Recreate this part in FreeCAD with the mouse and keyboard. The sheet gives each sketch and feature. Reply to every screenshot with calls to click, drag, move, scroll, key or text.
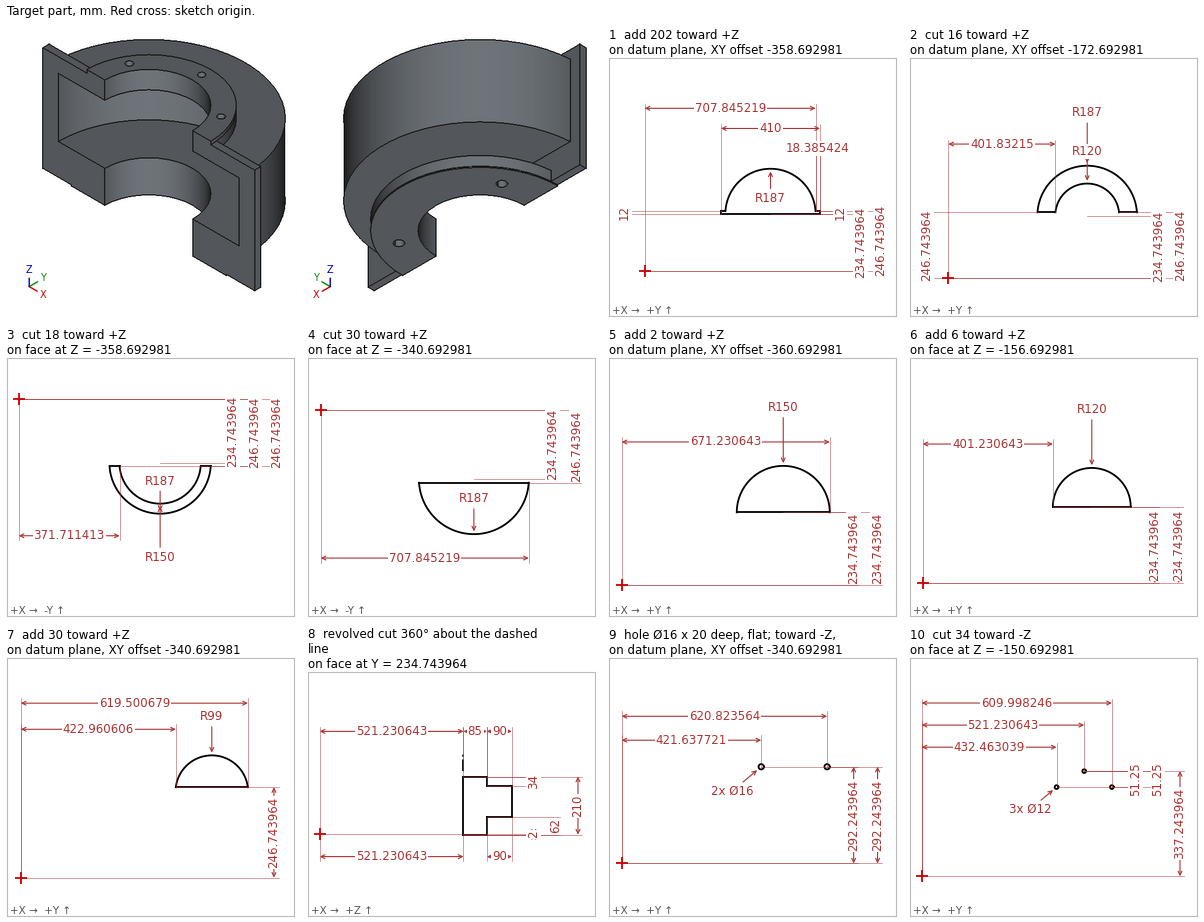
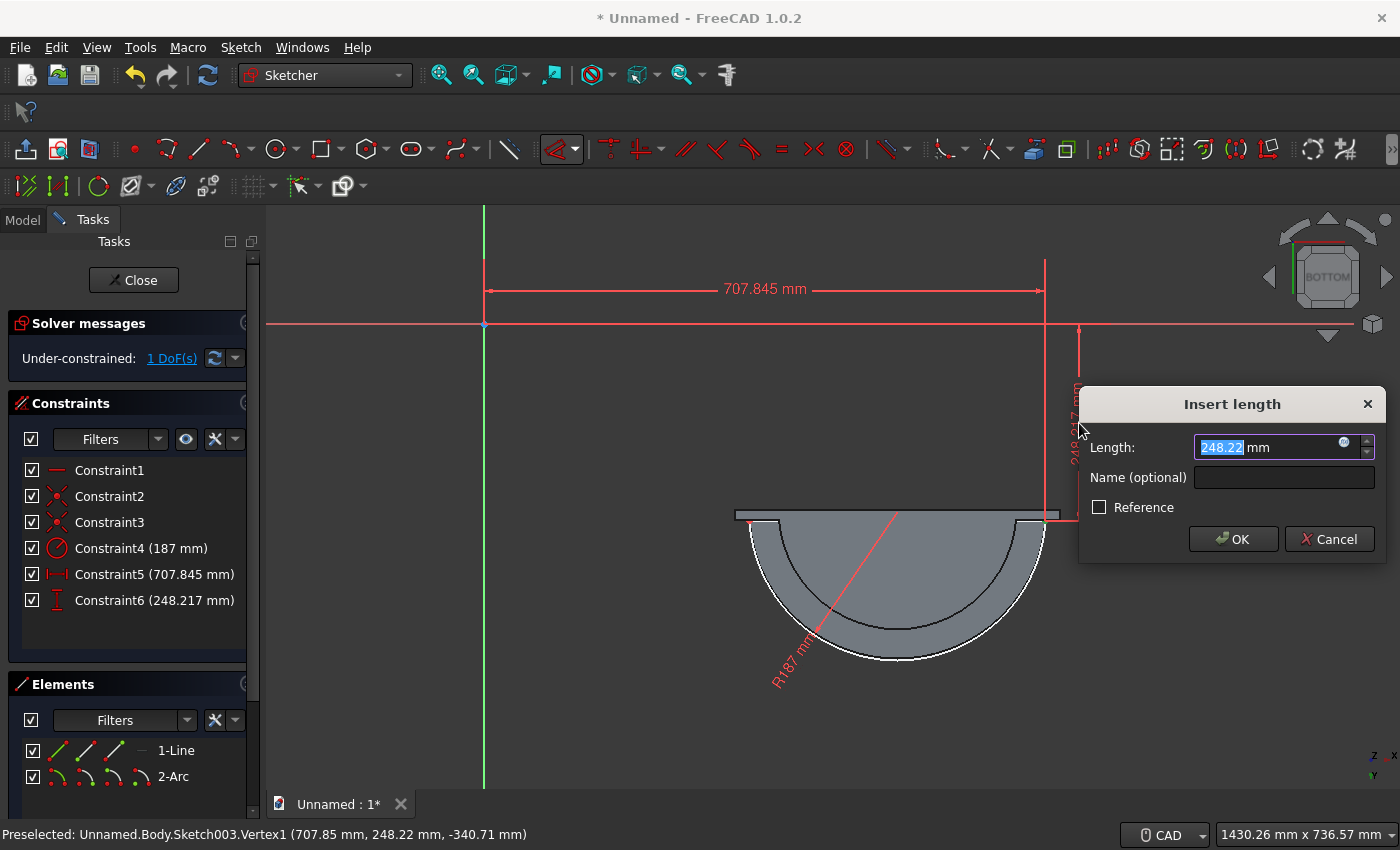
text(246.743964)
key(Return)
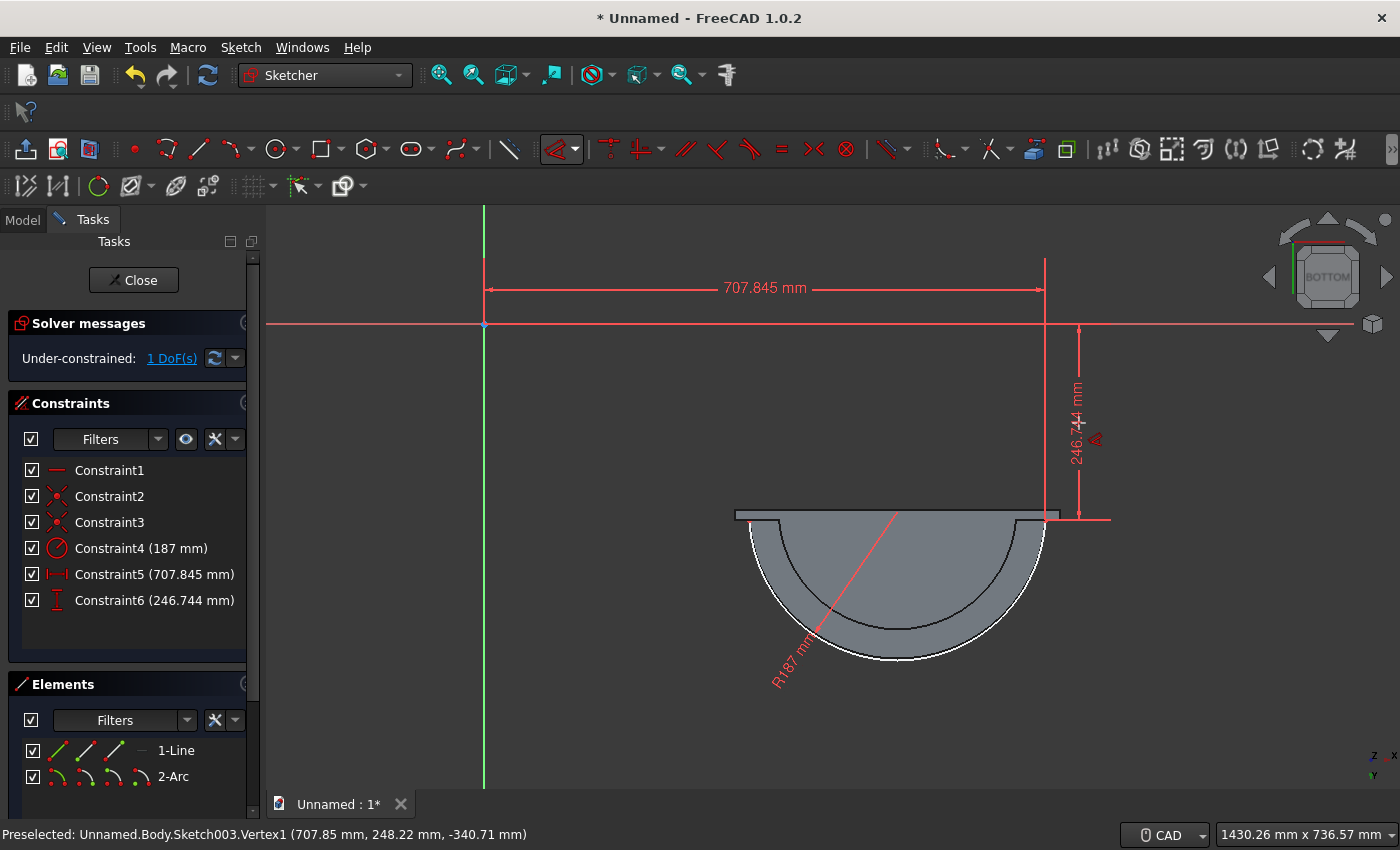
click(897, 512)
click(450, 418)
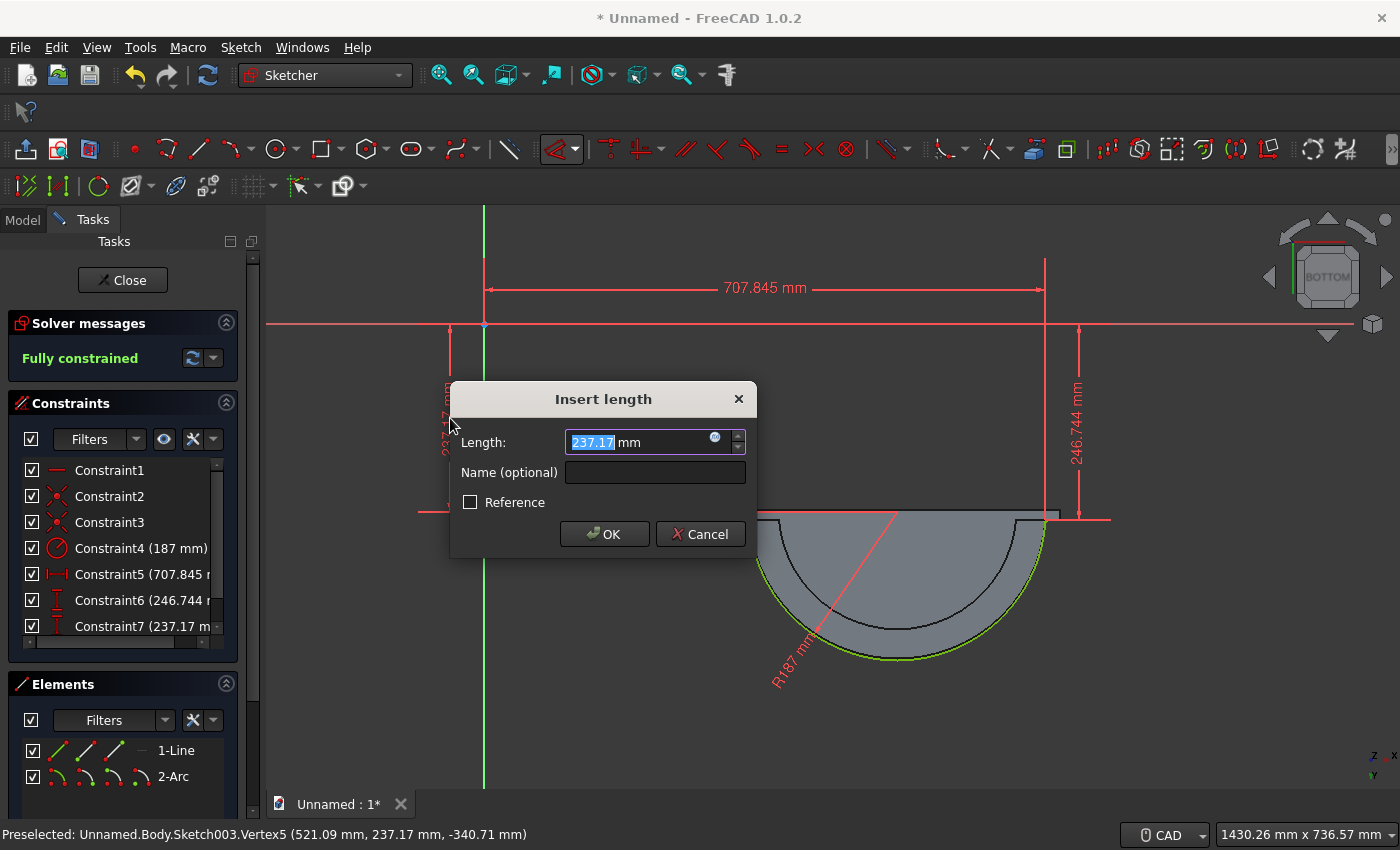
text(234.743964)
key(Return)
key(Escape)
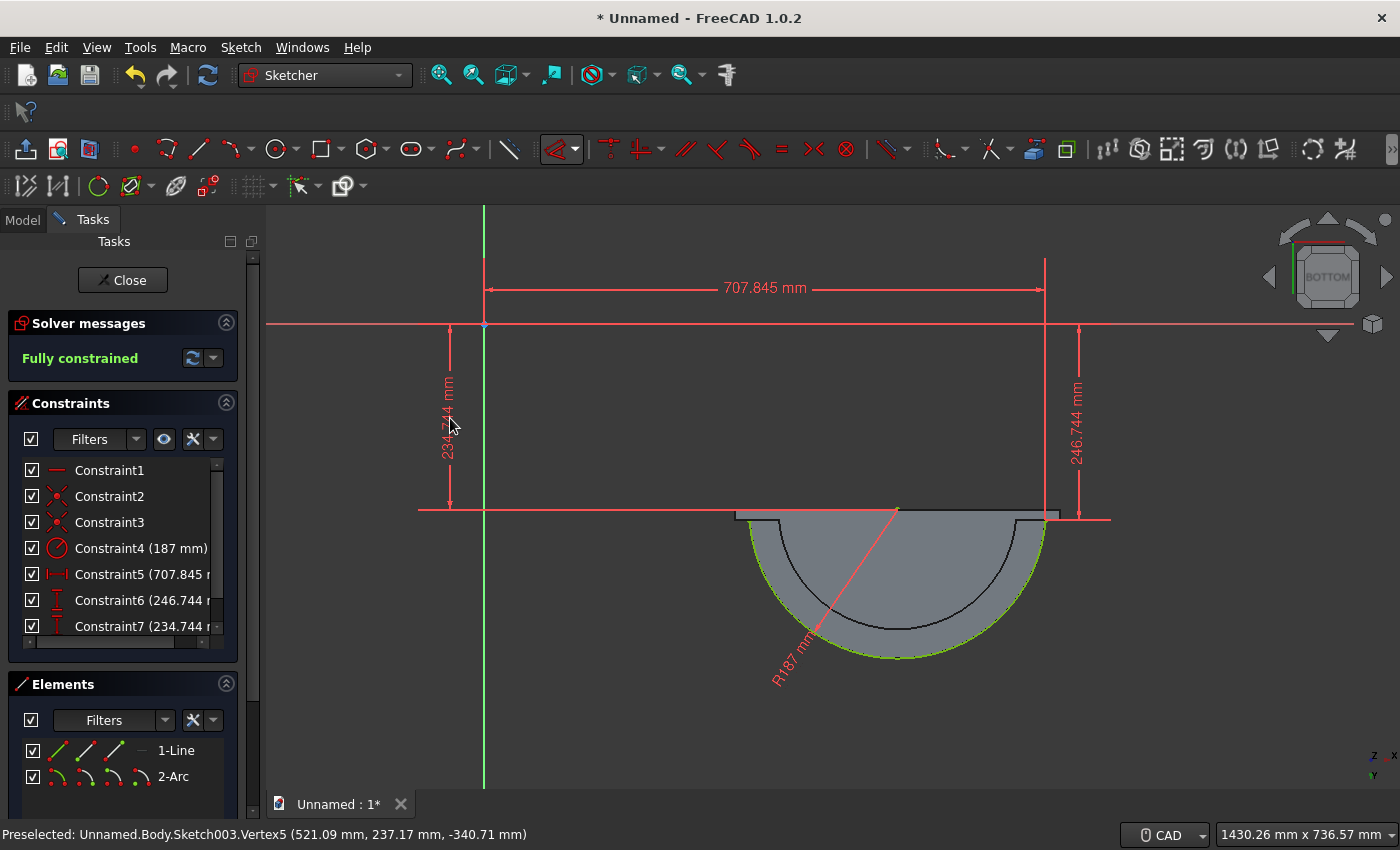
click(123, 280)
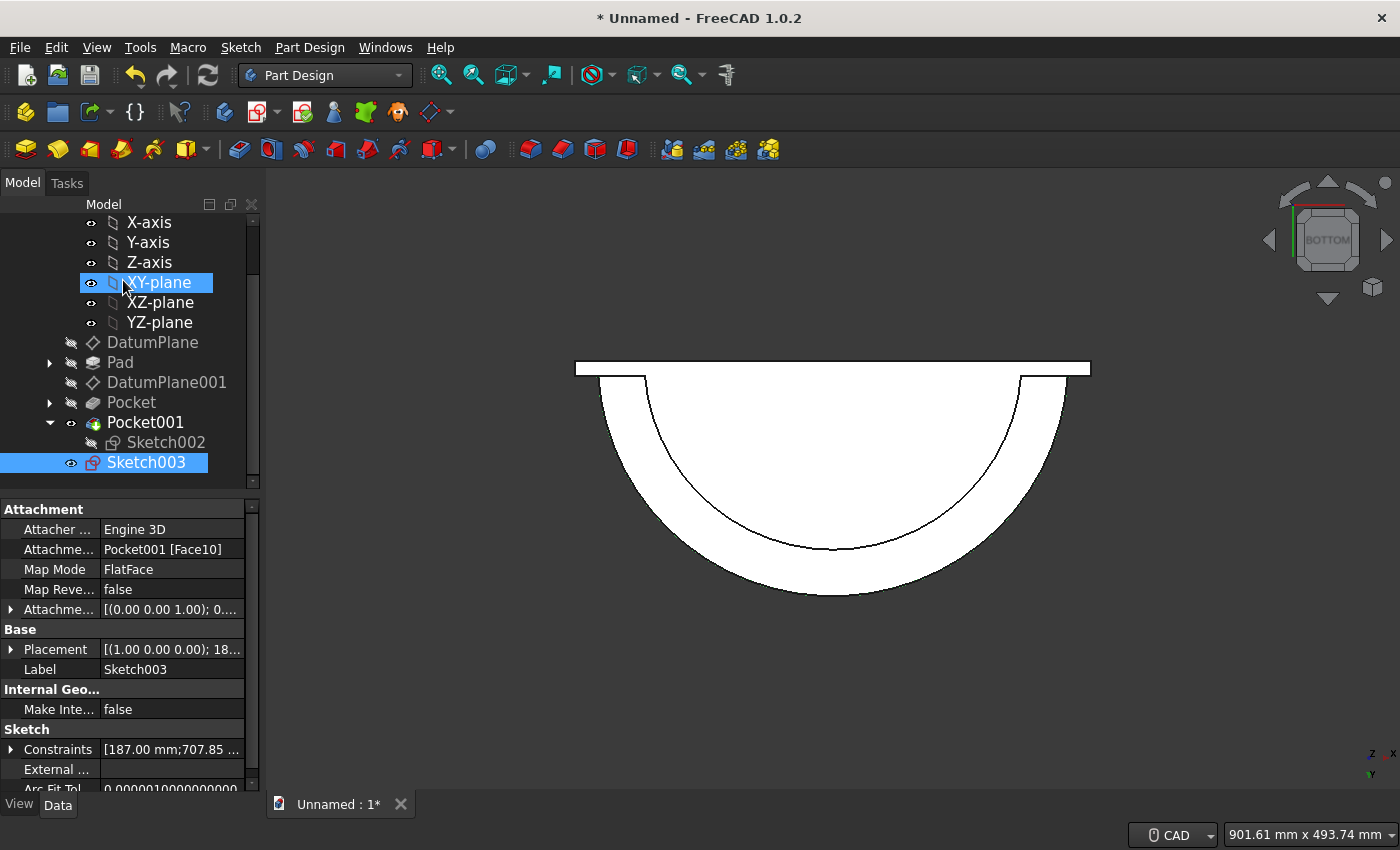
click(240, 150)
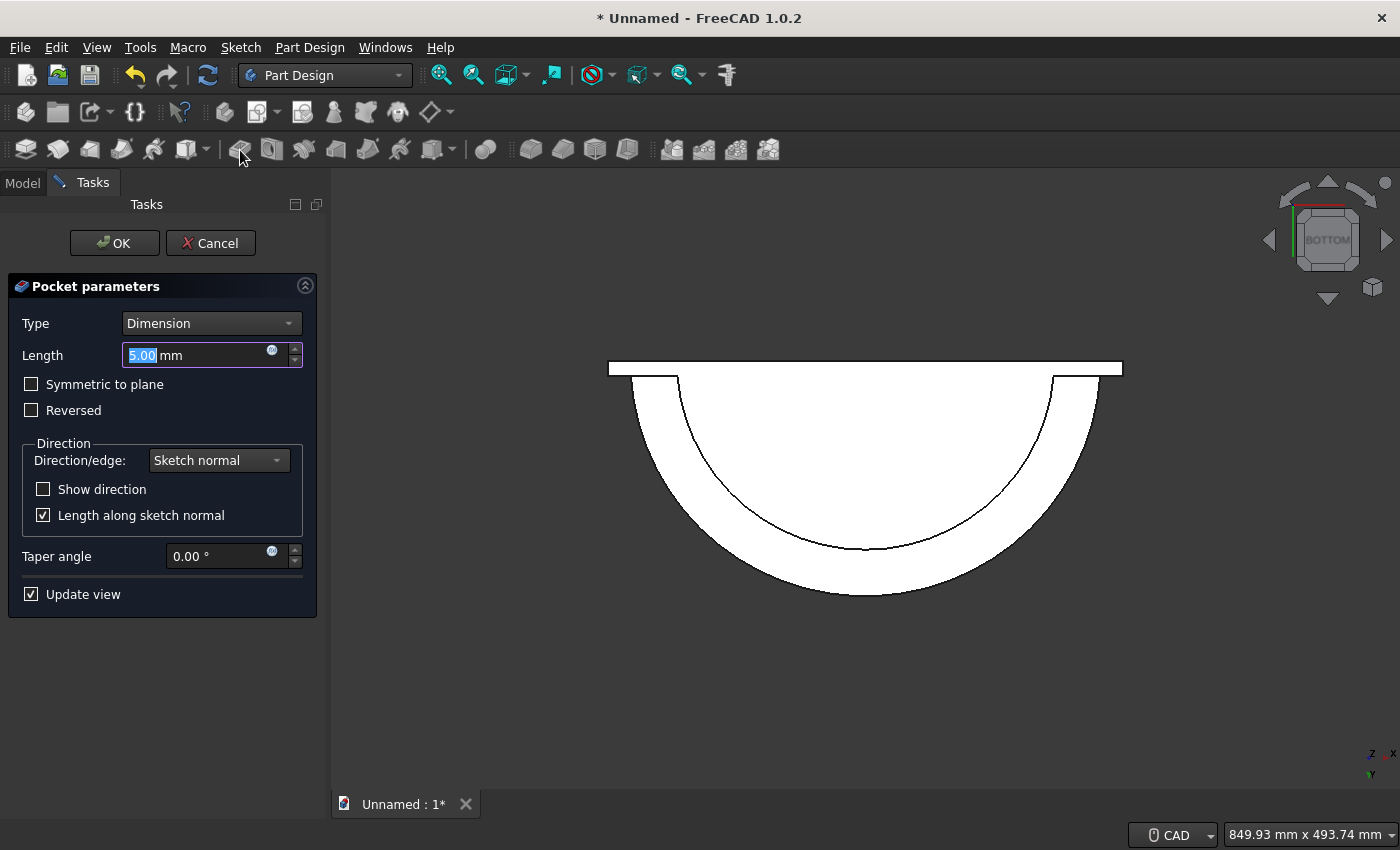
text(30)
key(Tab)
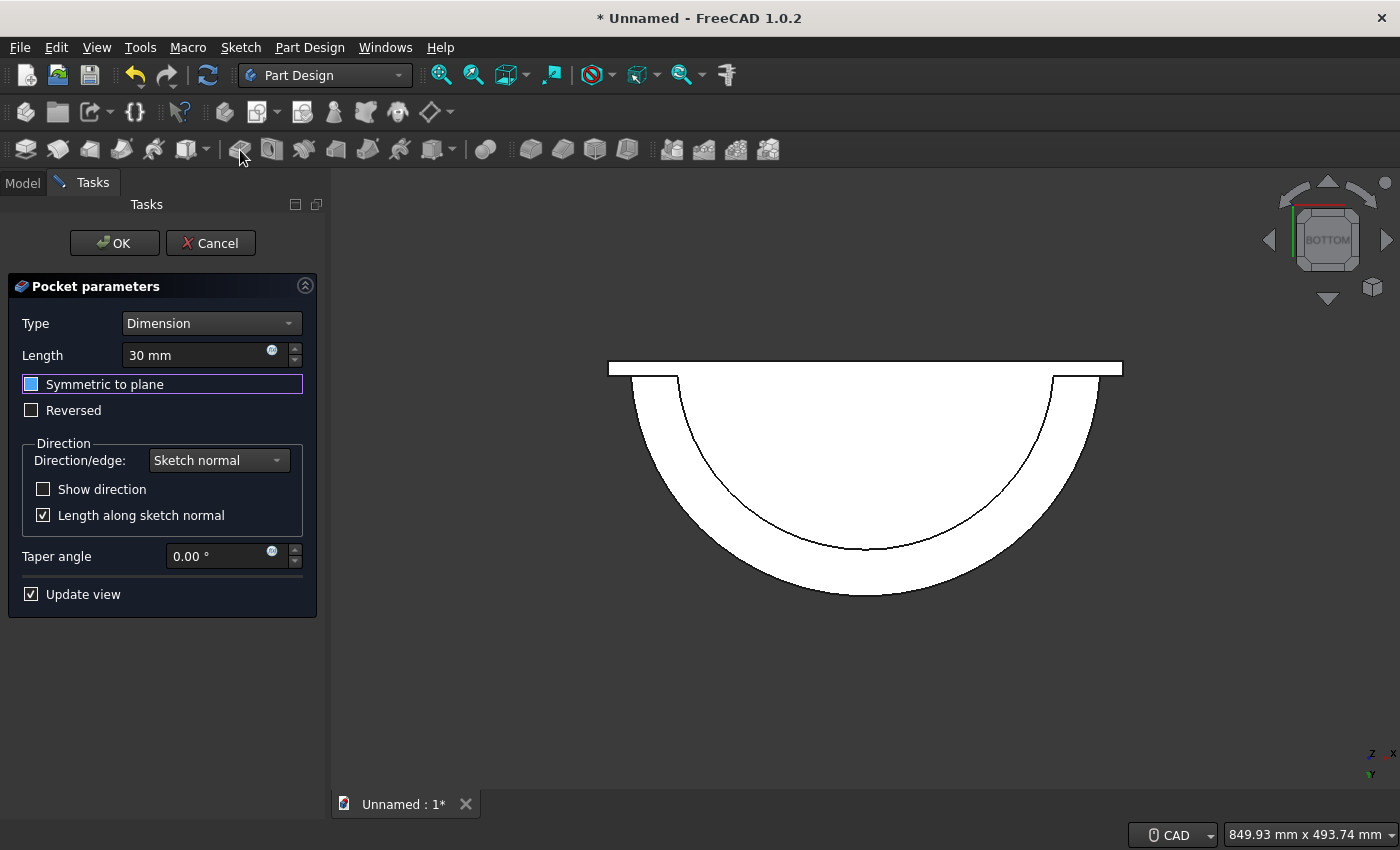
click(115, 243)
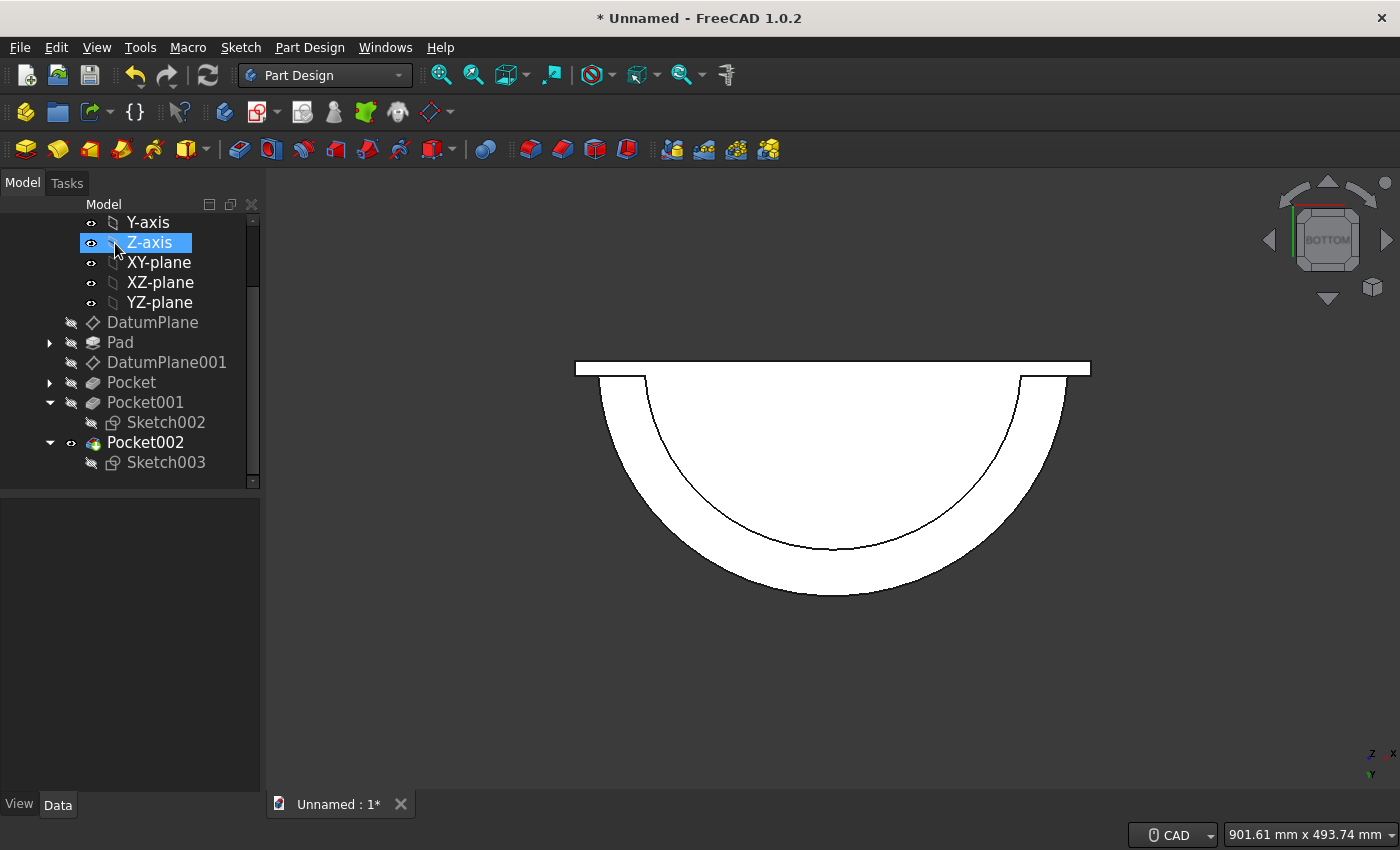
scroll(160, 338, down, 3)